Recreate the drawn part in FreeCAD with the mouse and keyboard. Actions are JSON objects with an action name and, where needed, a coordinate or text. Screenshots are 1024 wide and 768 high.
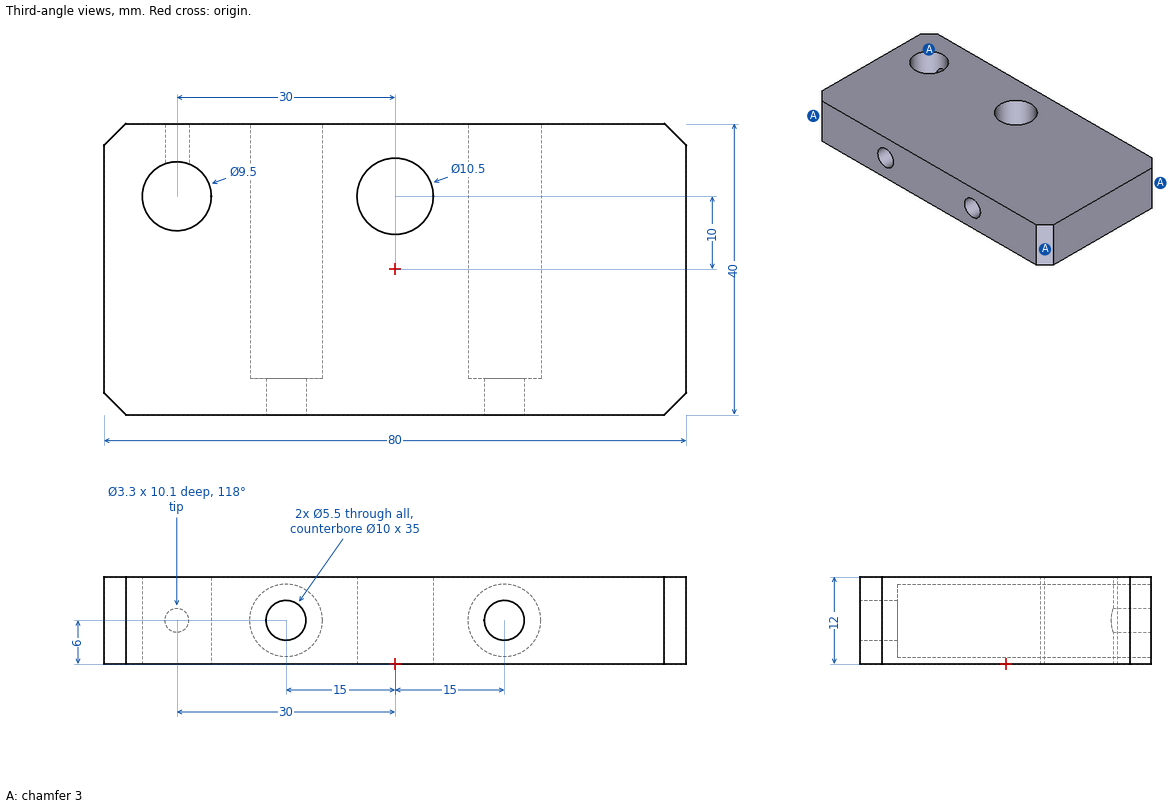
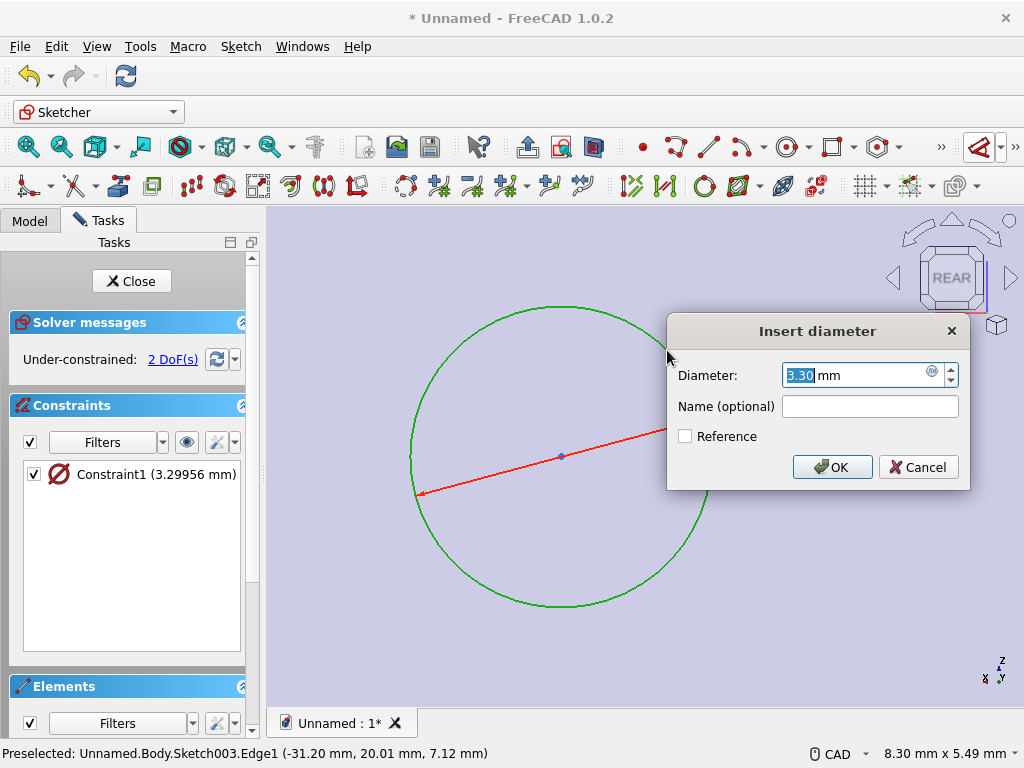
{"action": "type", "text": "3.3"}
{"action": "key", "text": "Return"}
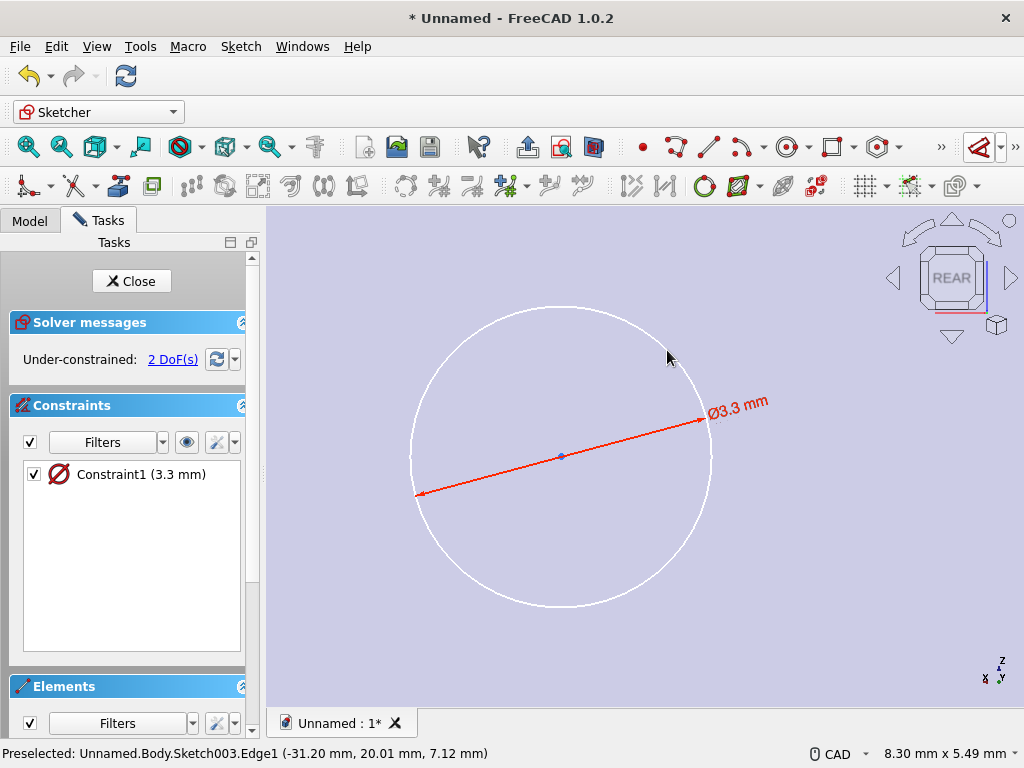
{"action": "left_click", "coordinate": [561, 457]}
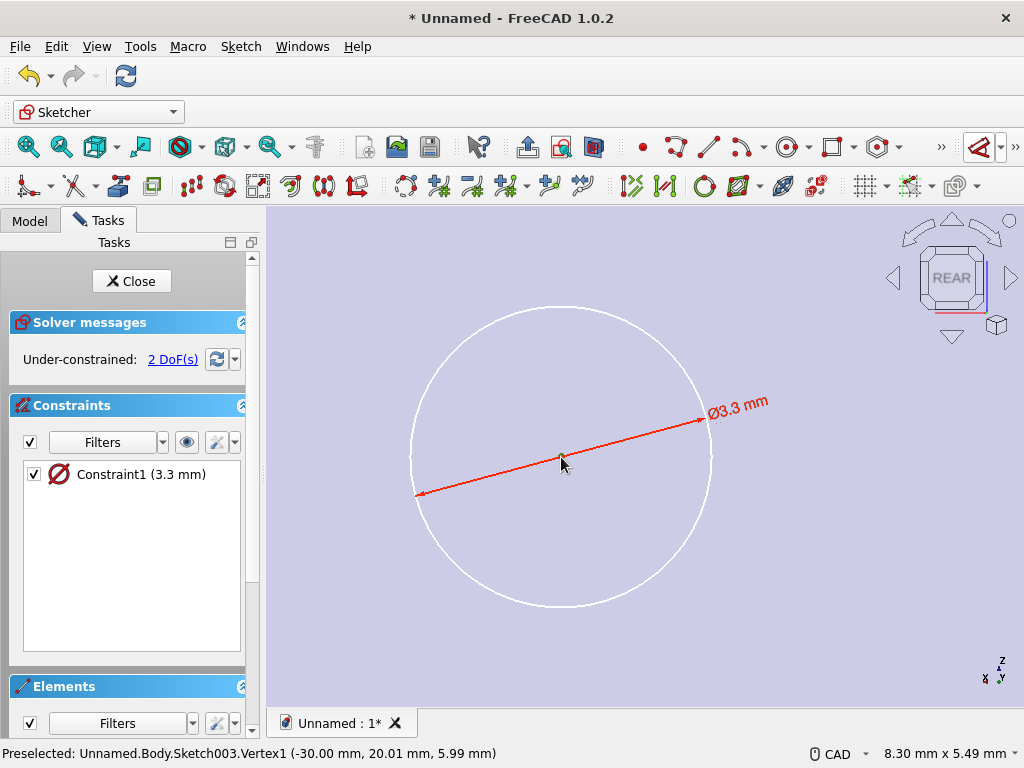
{"action": "key", "text": "i"}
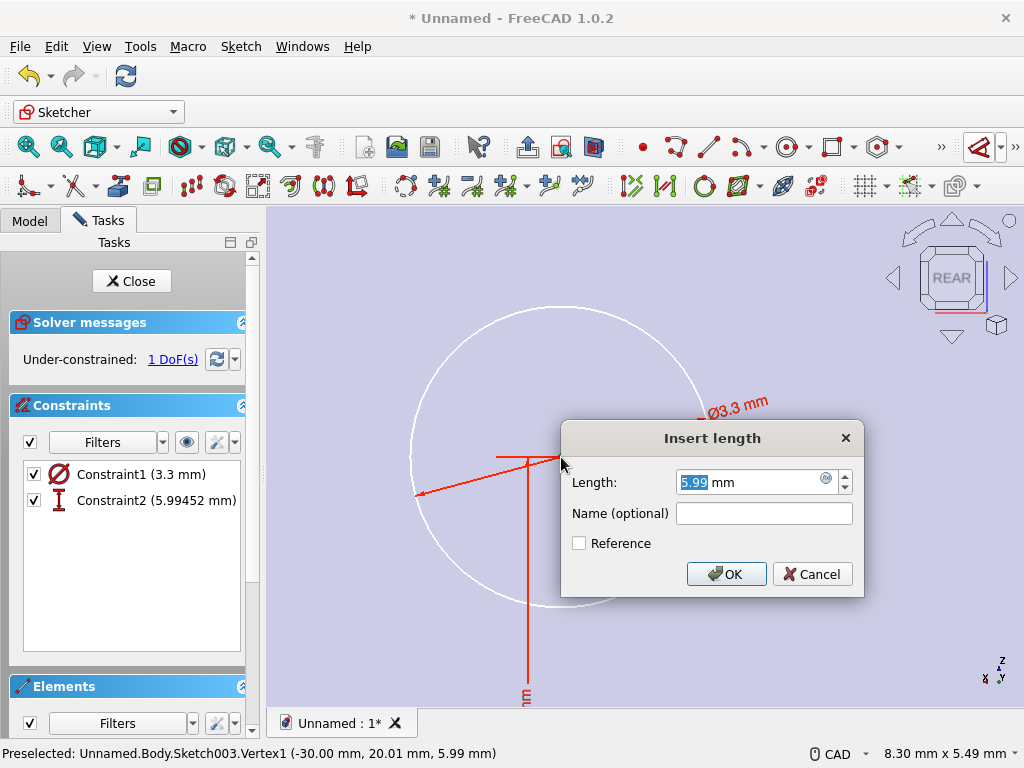
{"action": "type", "text": "6"}
{"action": "key", "text": "Return"}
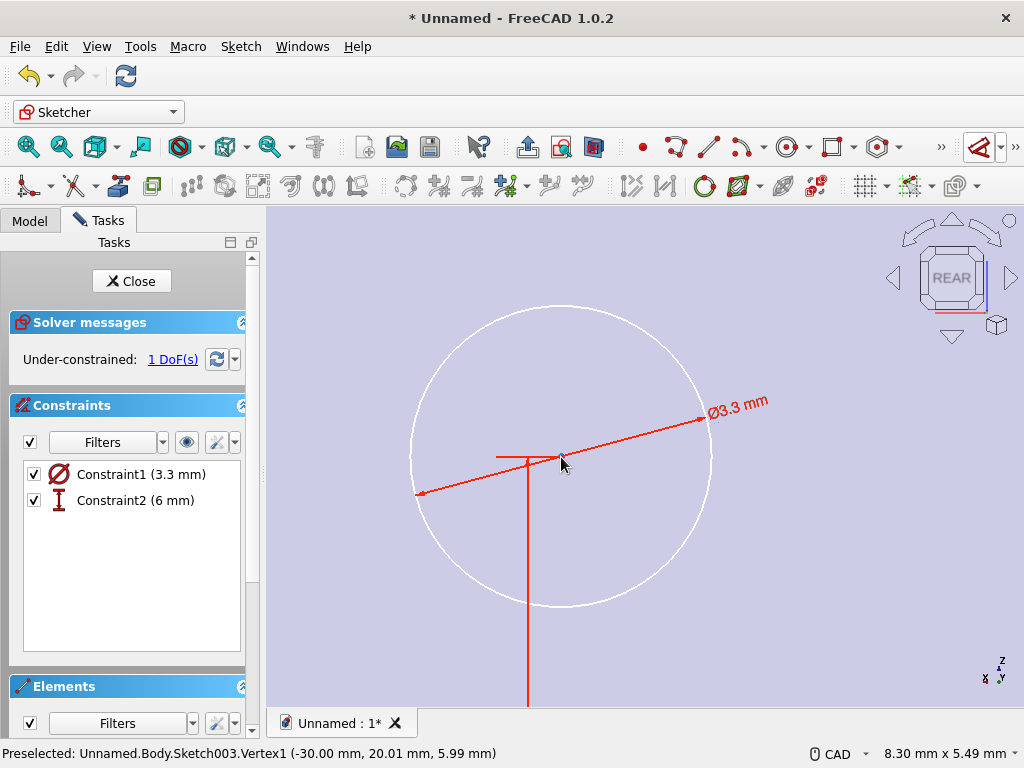
{"action": "left_click", "coordinate": [561, 456]}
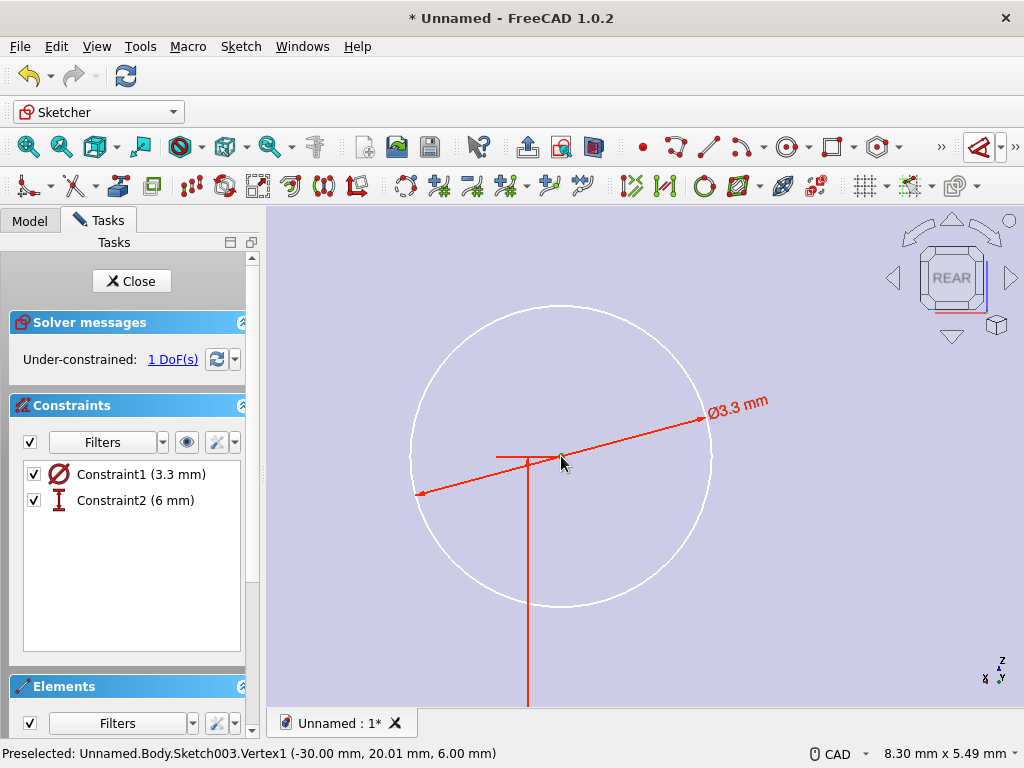
{"action": "key", "text": "l"}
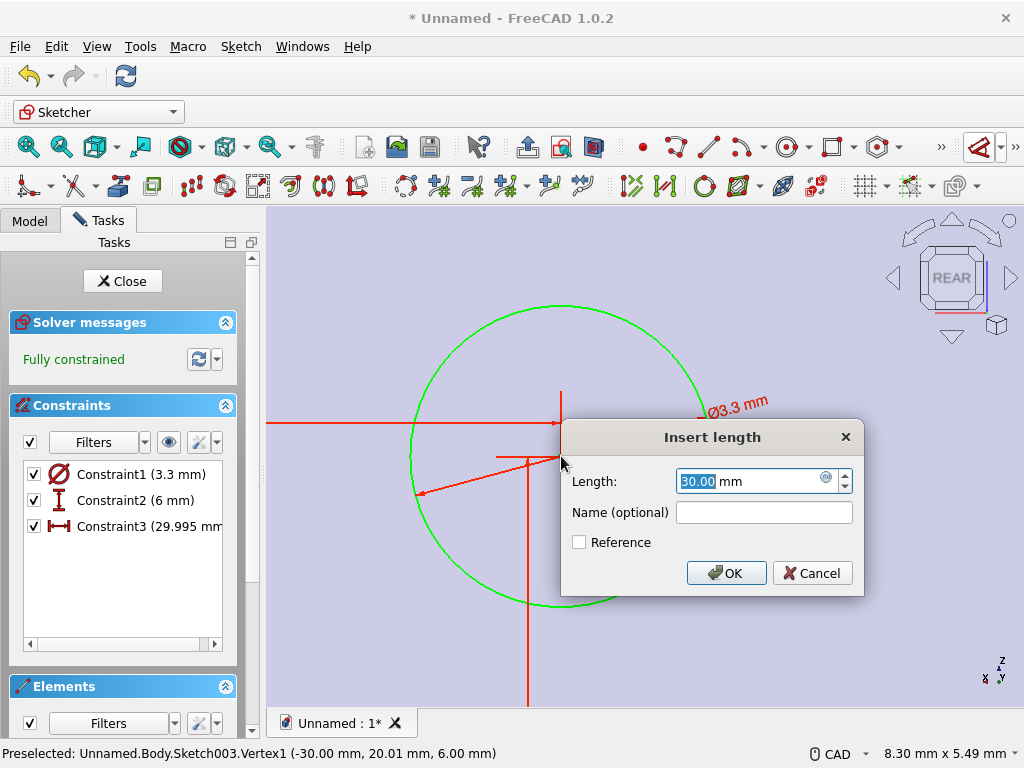
{"action": "type", "text": "30"}
{"action": "key", "text": "Return"}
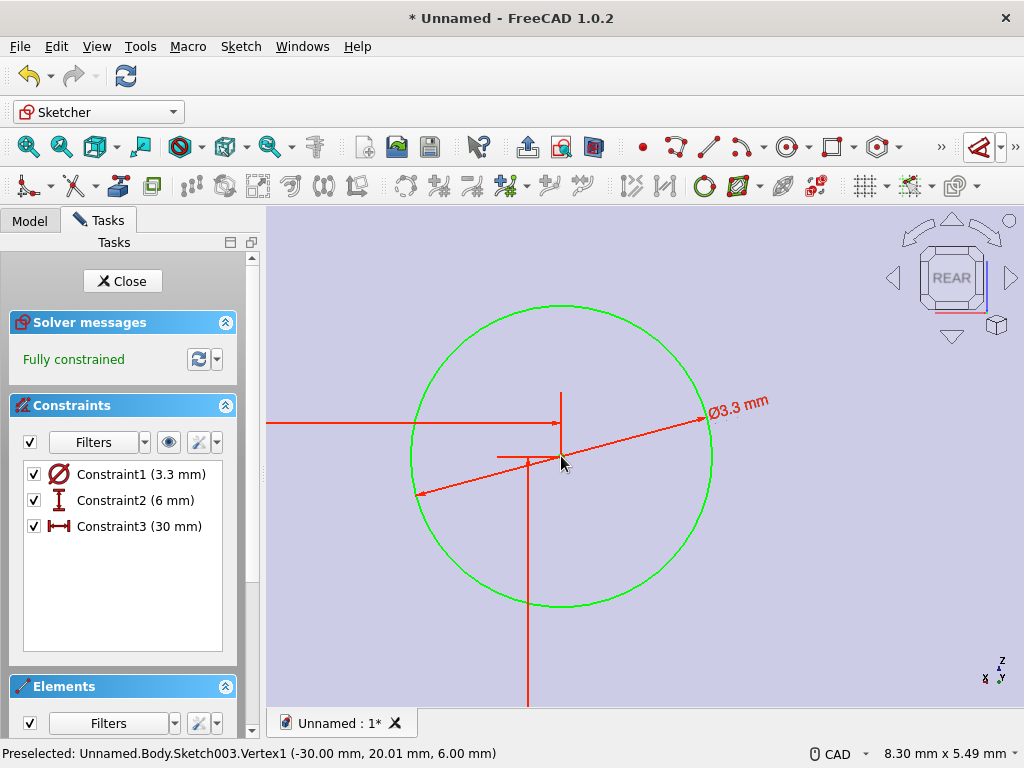
{"action": "left_click", "coordinate": [123, 281]}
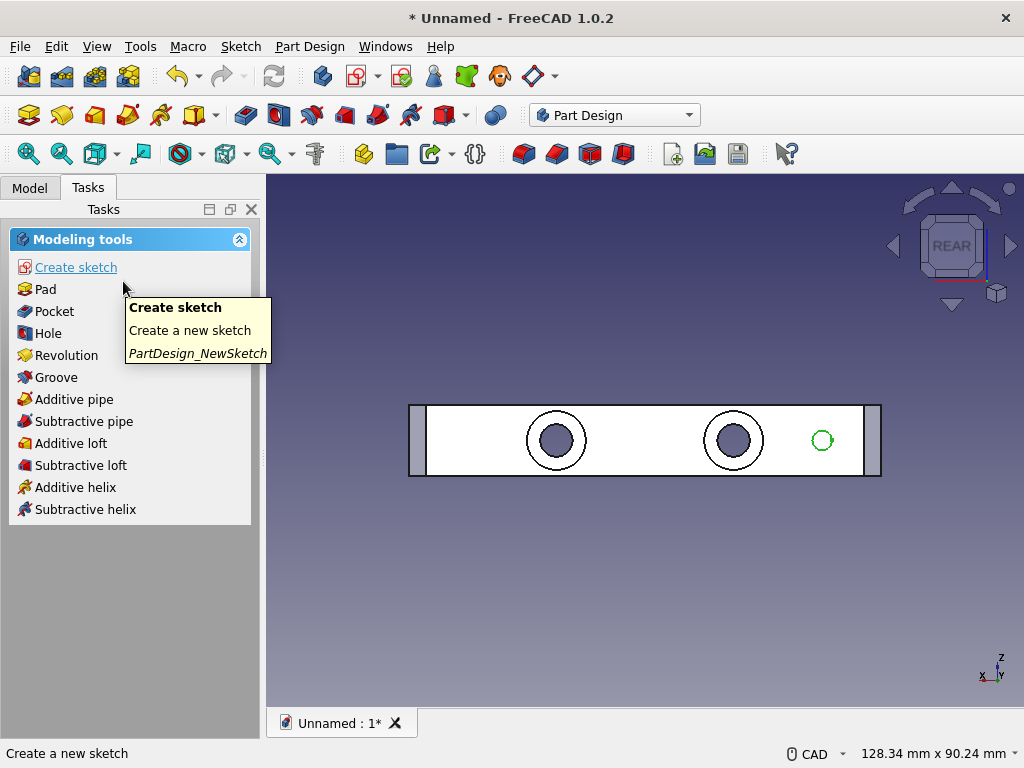
{"action": "left_click", "coordinate": [279, 116]}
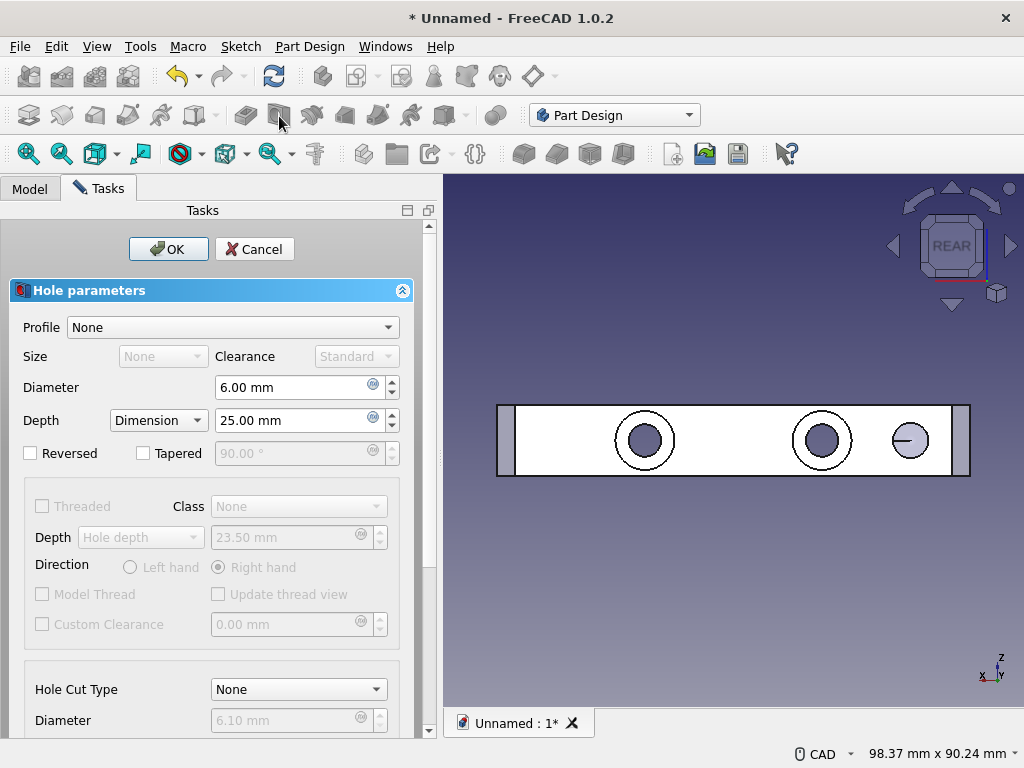
{"action": "triple_click", "coordinate": [300, 388]}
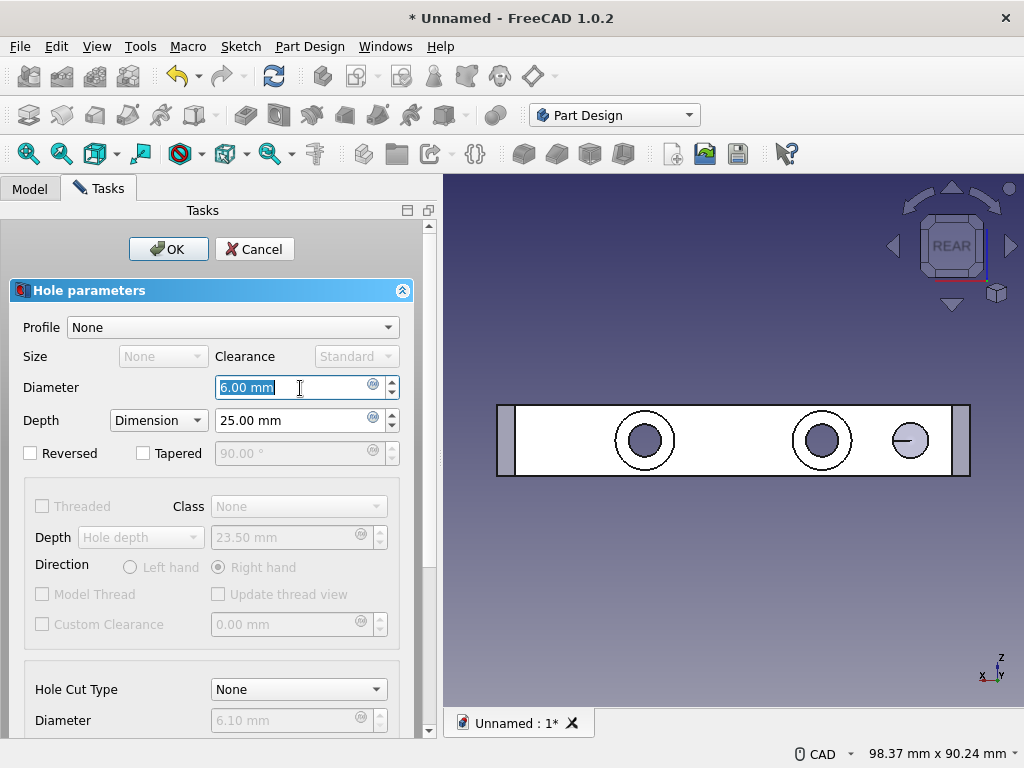
{"action": "type", "text": "3.3"}
{"action": "key", "text": "Tab"}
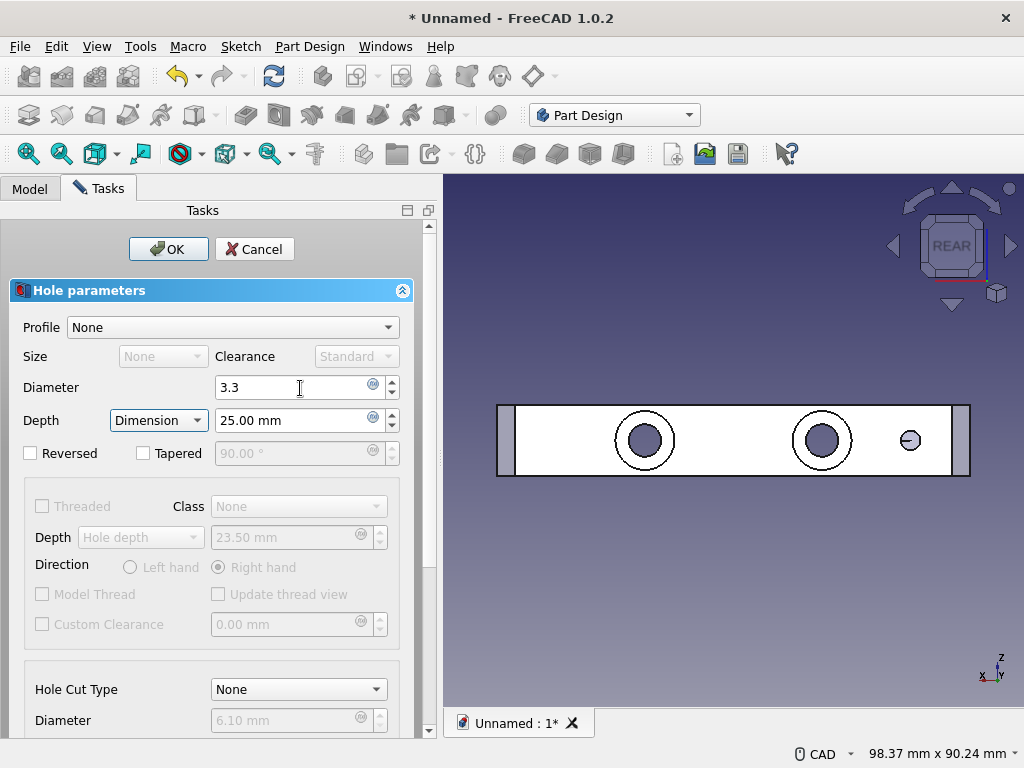
{"action": "triple_click", "coordinate": [300, 420]}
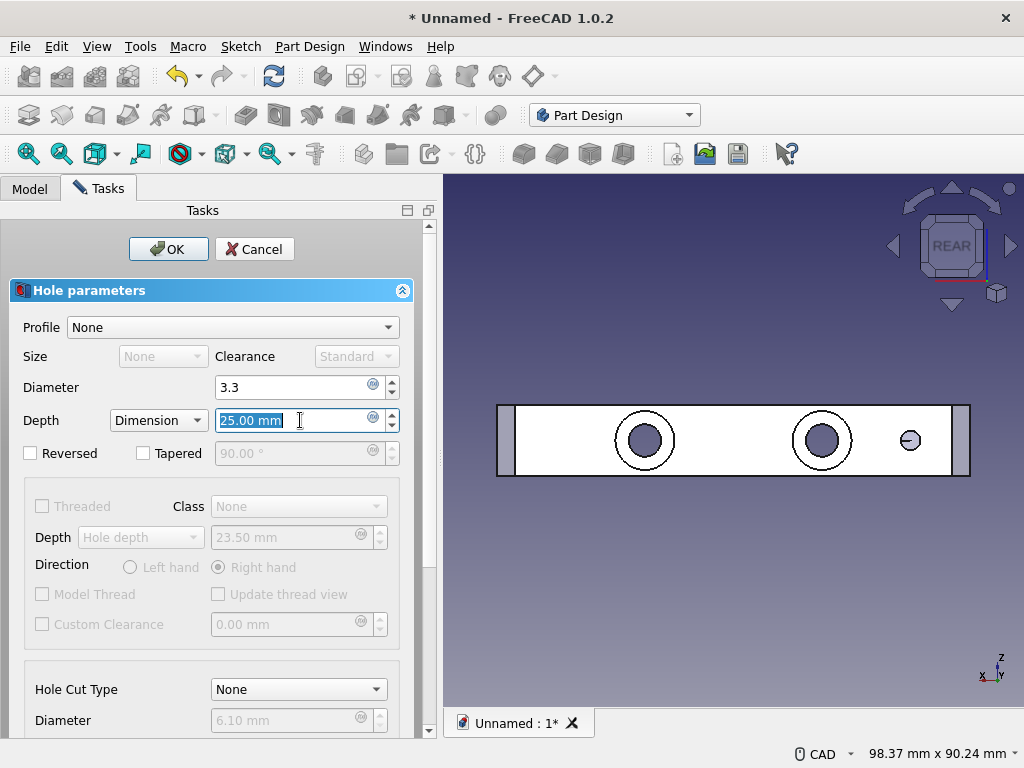
{"action": "type", "text": "10.1"}
{"action": "key", "text": "Tab"}